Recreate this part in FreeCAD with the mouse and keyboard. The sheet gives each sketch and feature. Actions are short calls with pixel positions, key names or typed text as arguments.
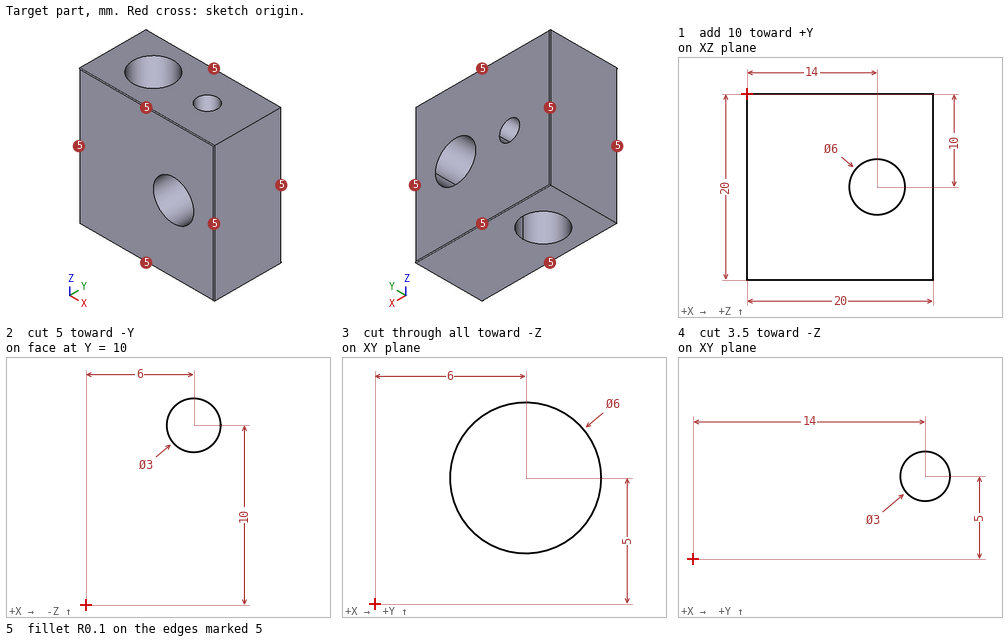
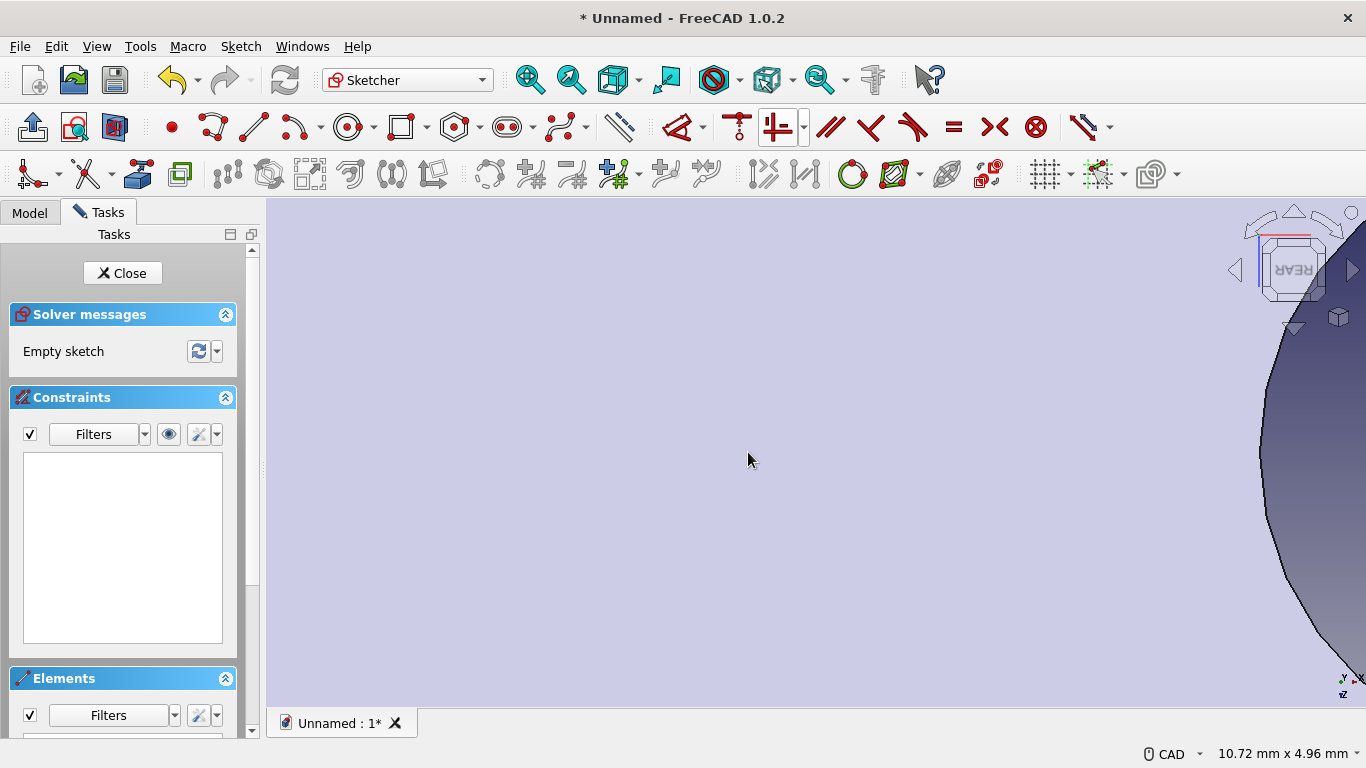
click(348, 128)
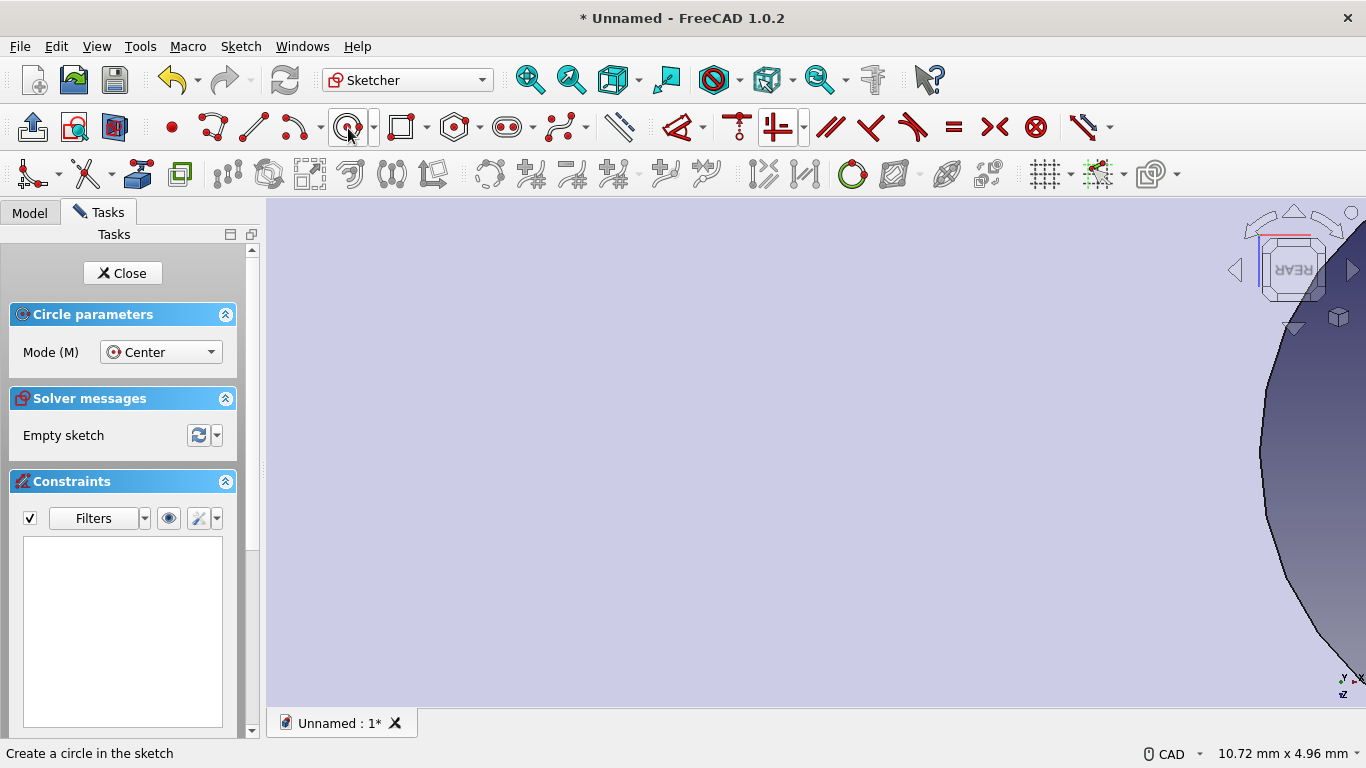
click(747, 452)
click(855, 344)
key(Escape)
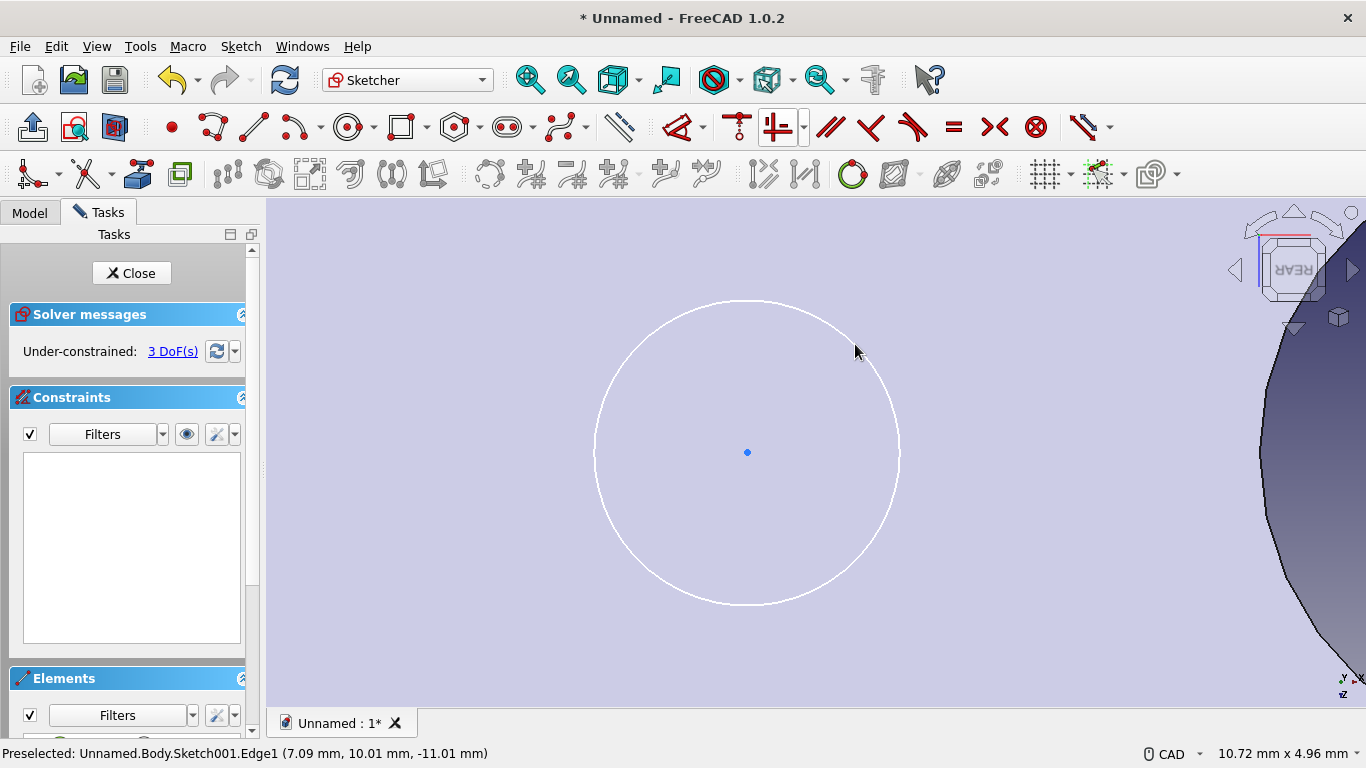
click(676, 128)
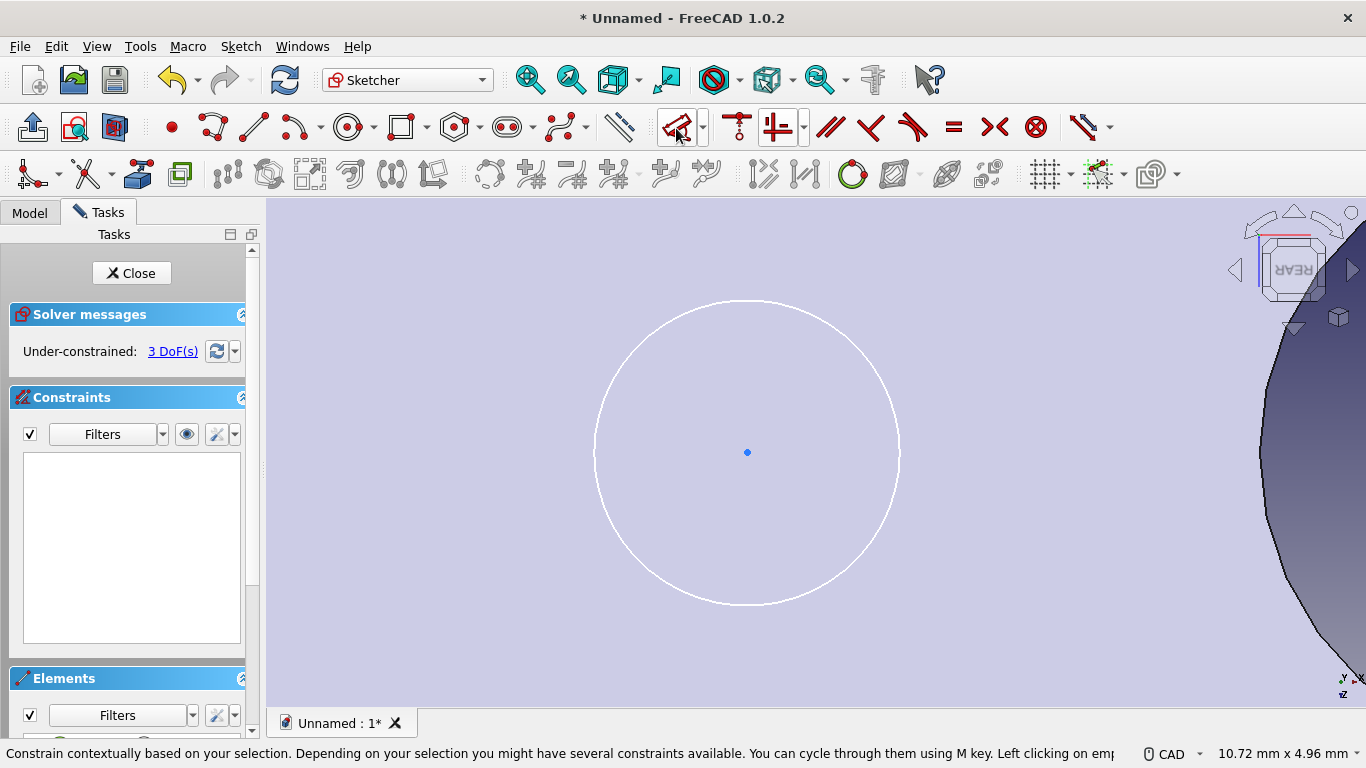
click(855, 345)
click(878, 322)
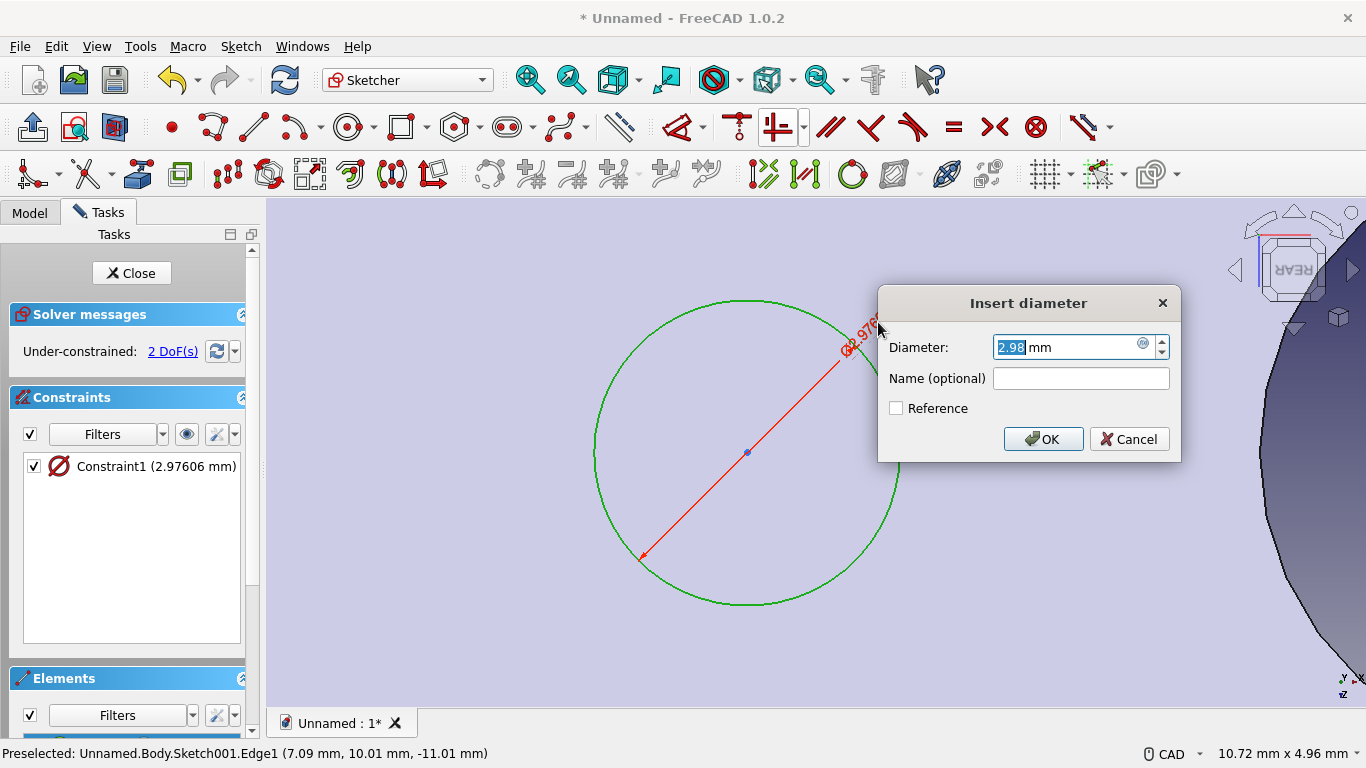
text(3)
key(Return)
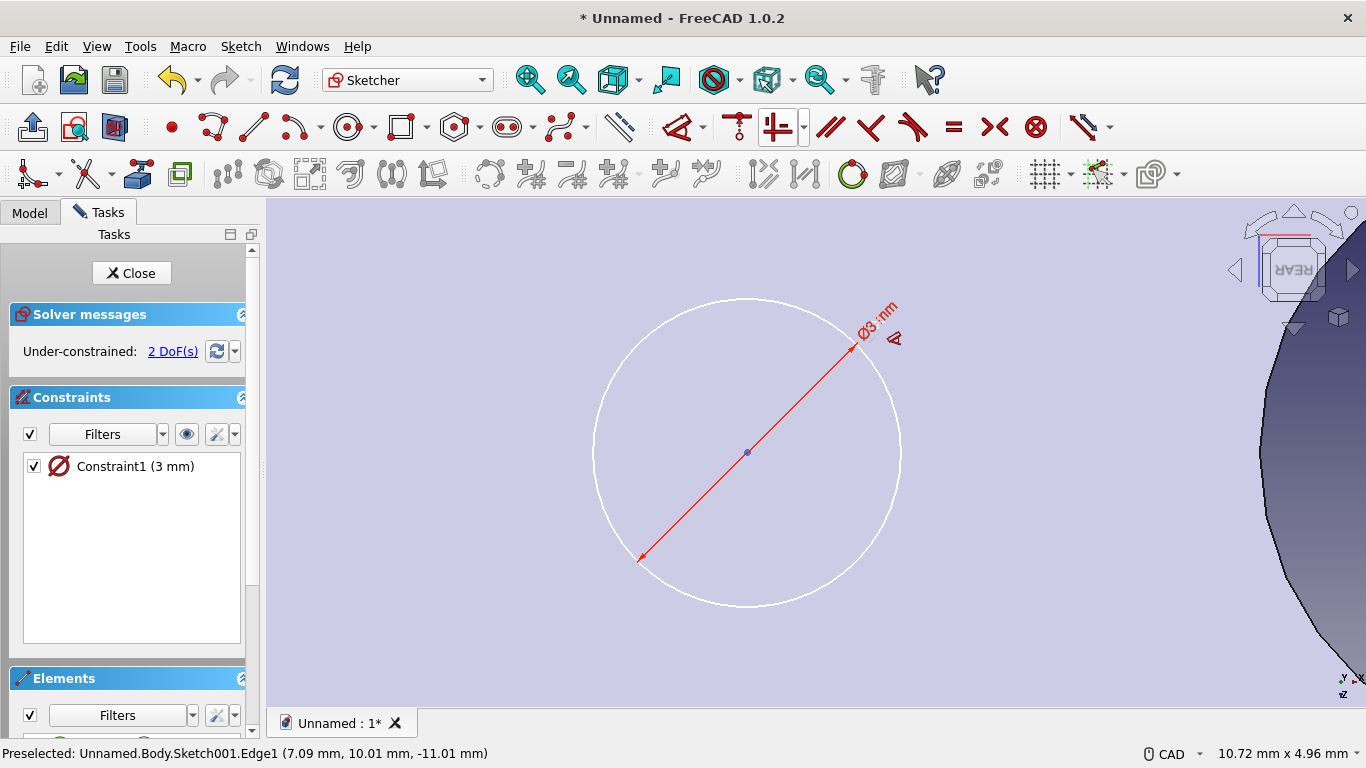
click(747, 453)
click(520, 419)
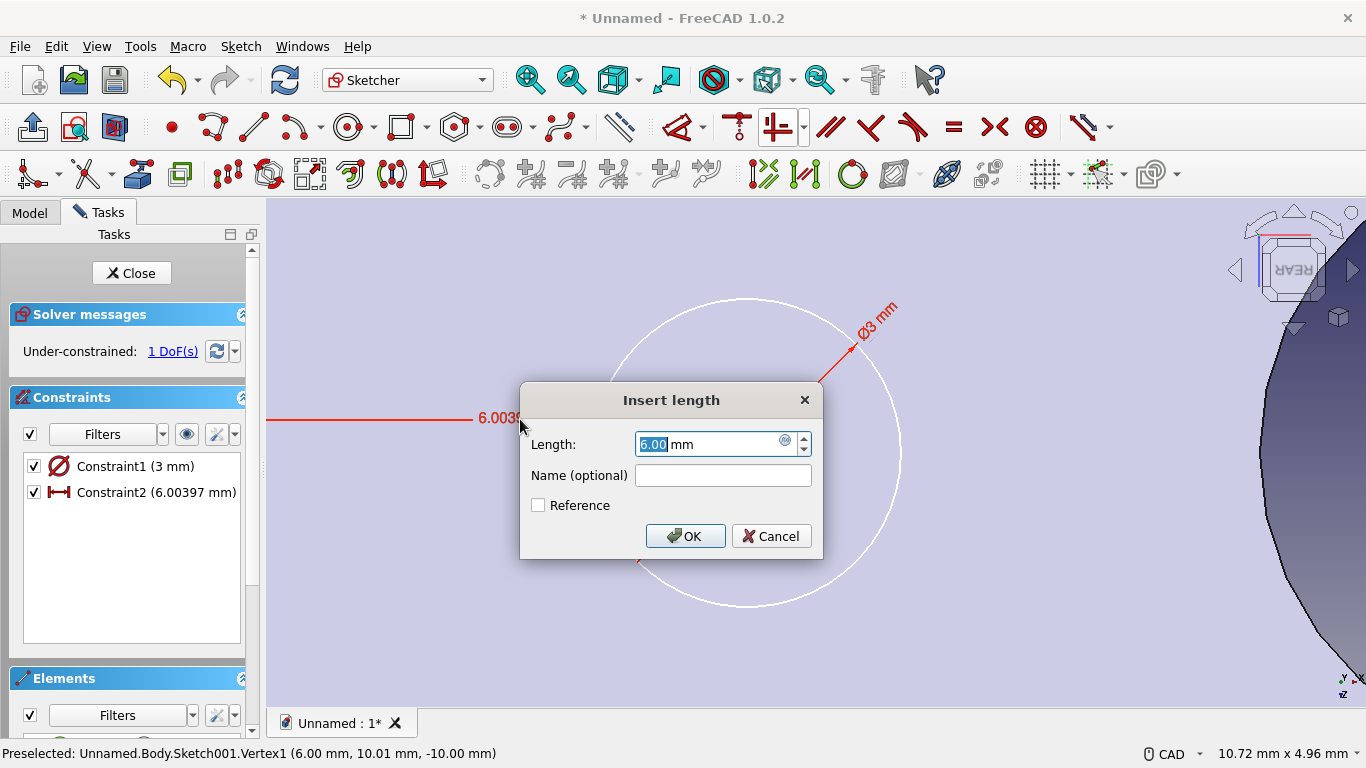
text(6)
key(Return)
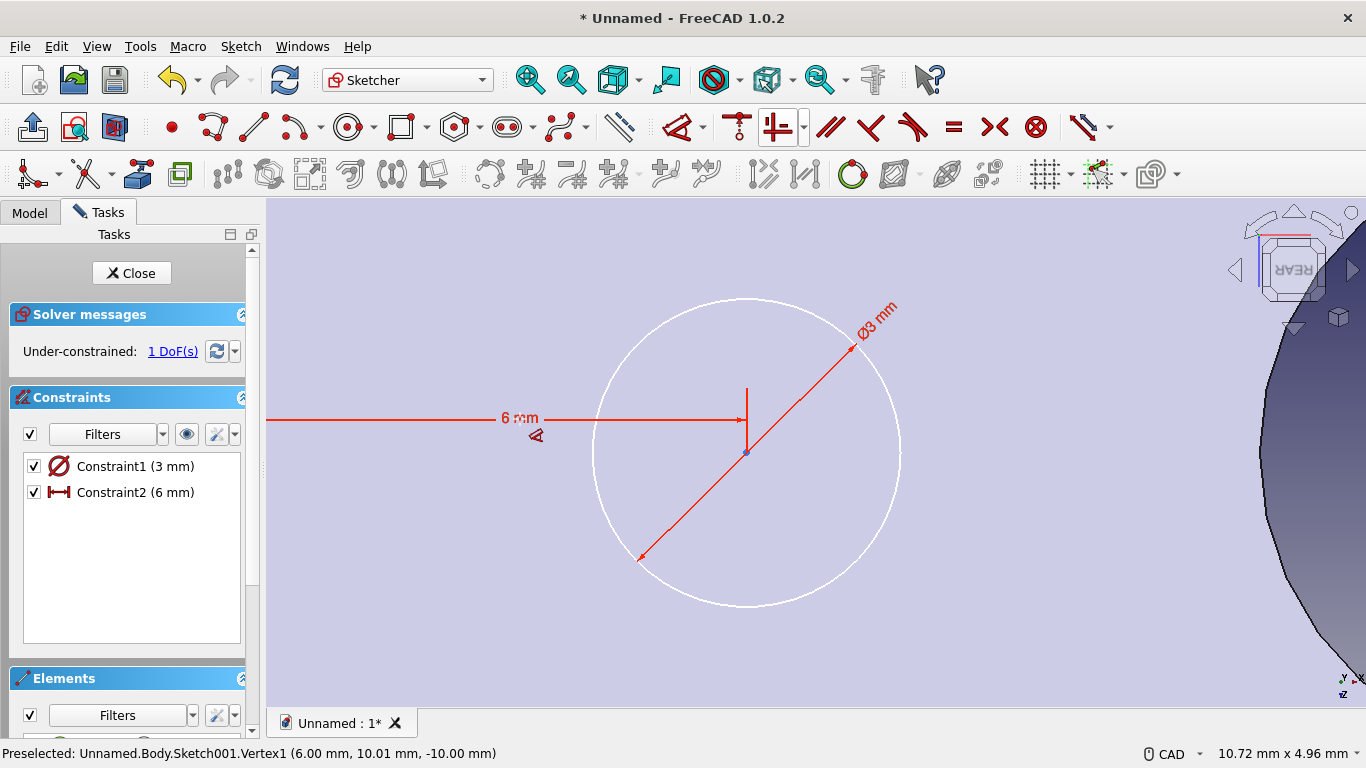
click(747, 453)
click(781, 566)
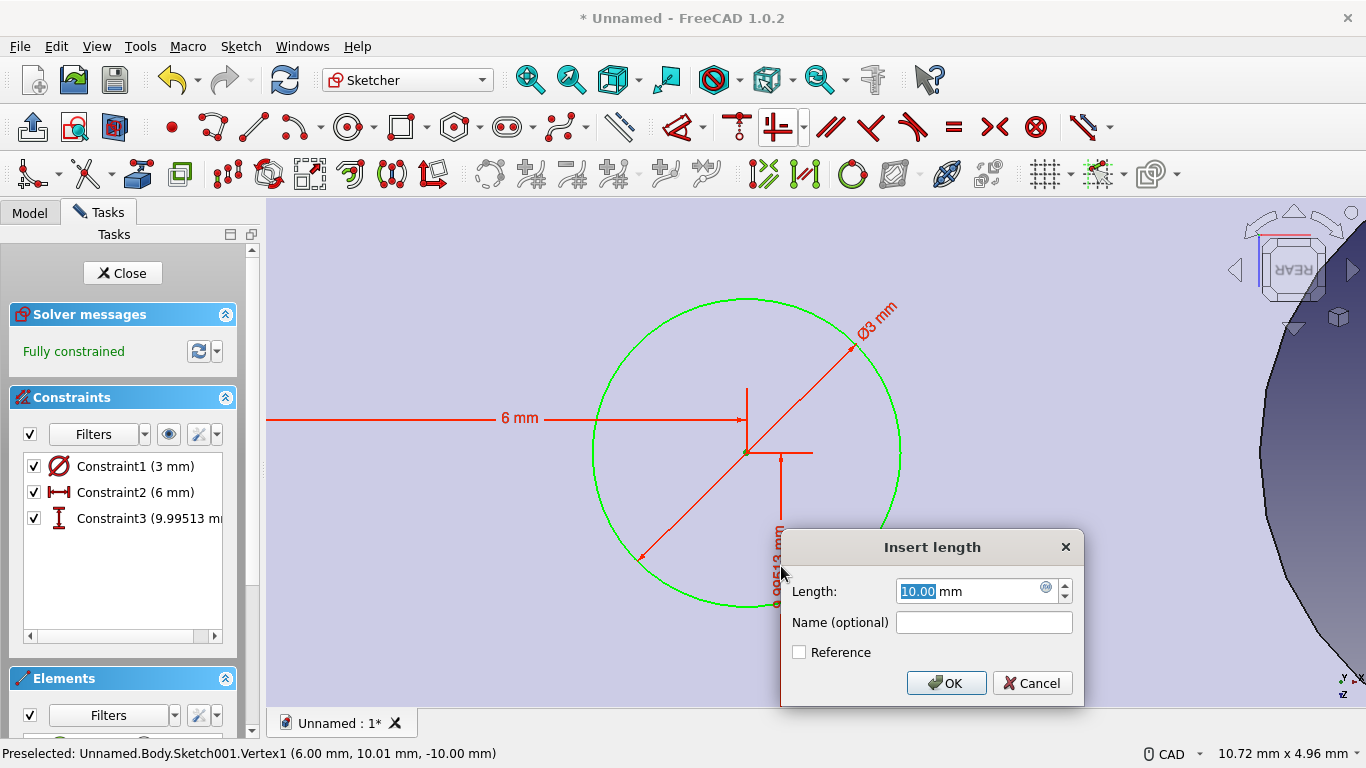
text(10)
key(Return)
key(Escape)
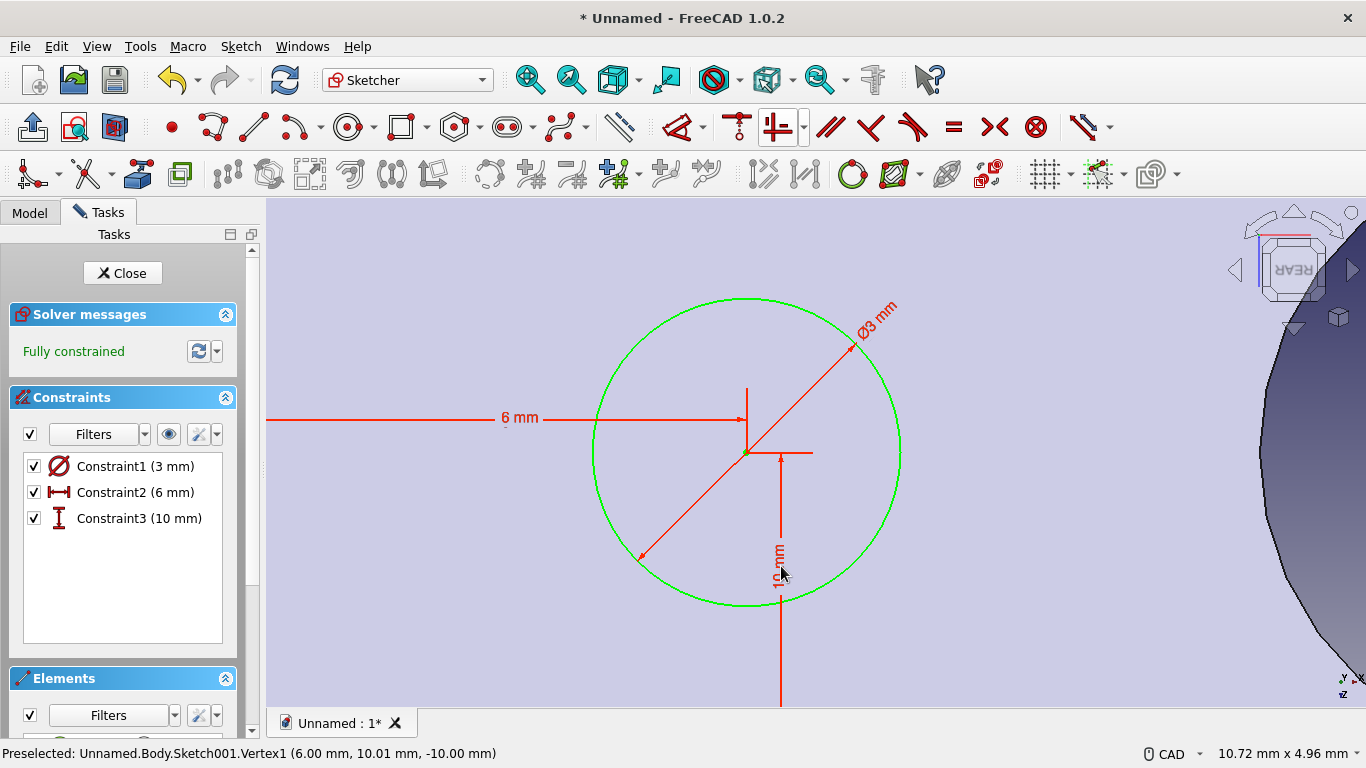
click(123, 273)